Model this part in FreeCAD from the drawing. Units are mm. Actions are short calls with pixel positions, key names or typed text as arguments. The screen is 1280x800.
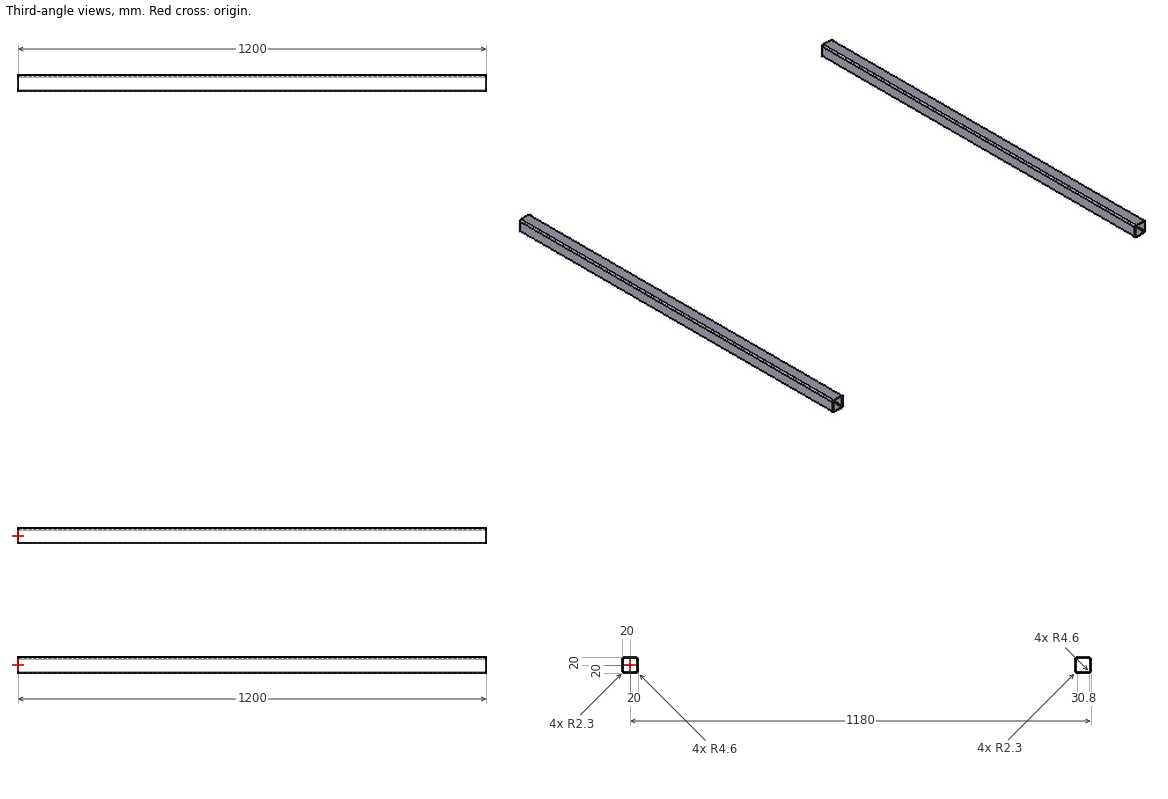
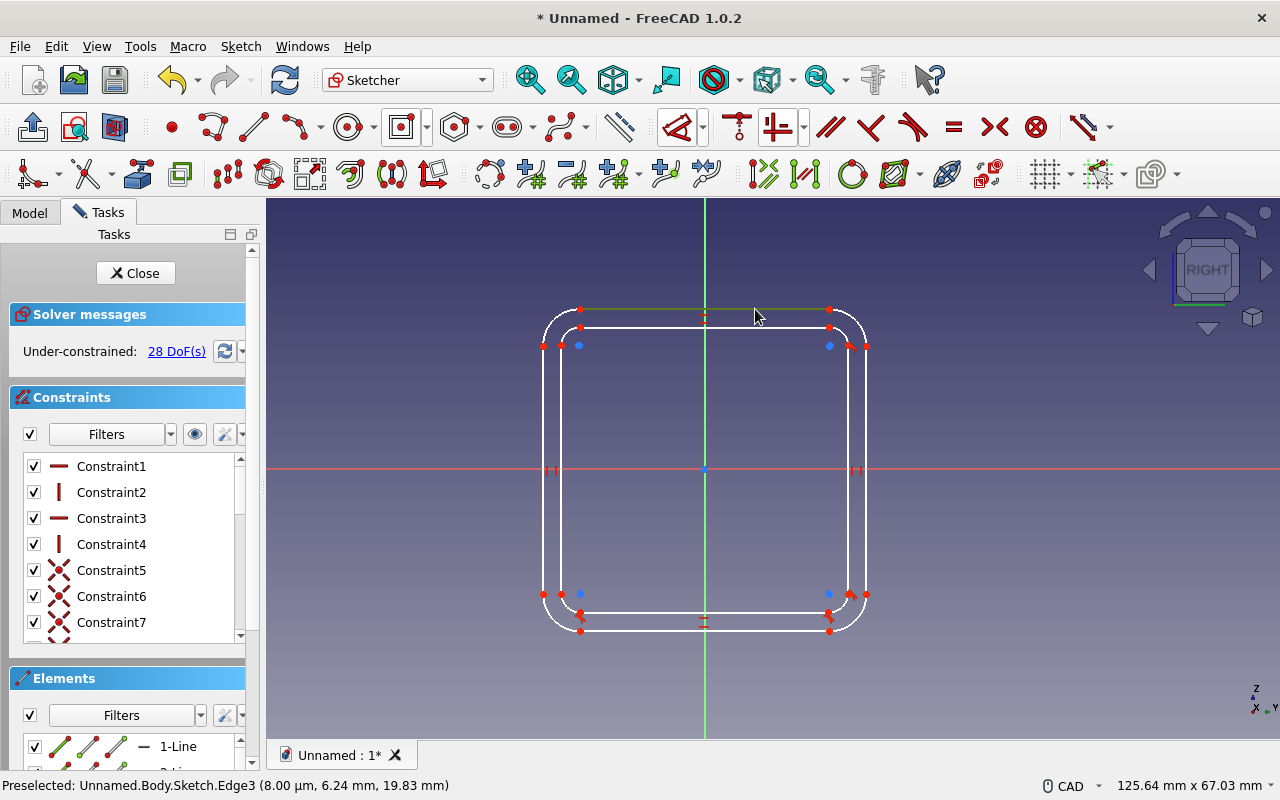
click(862, 330)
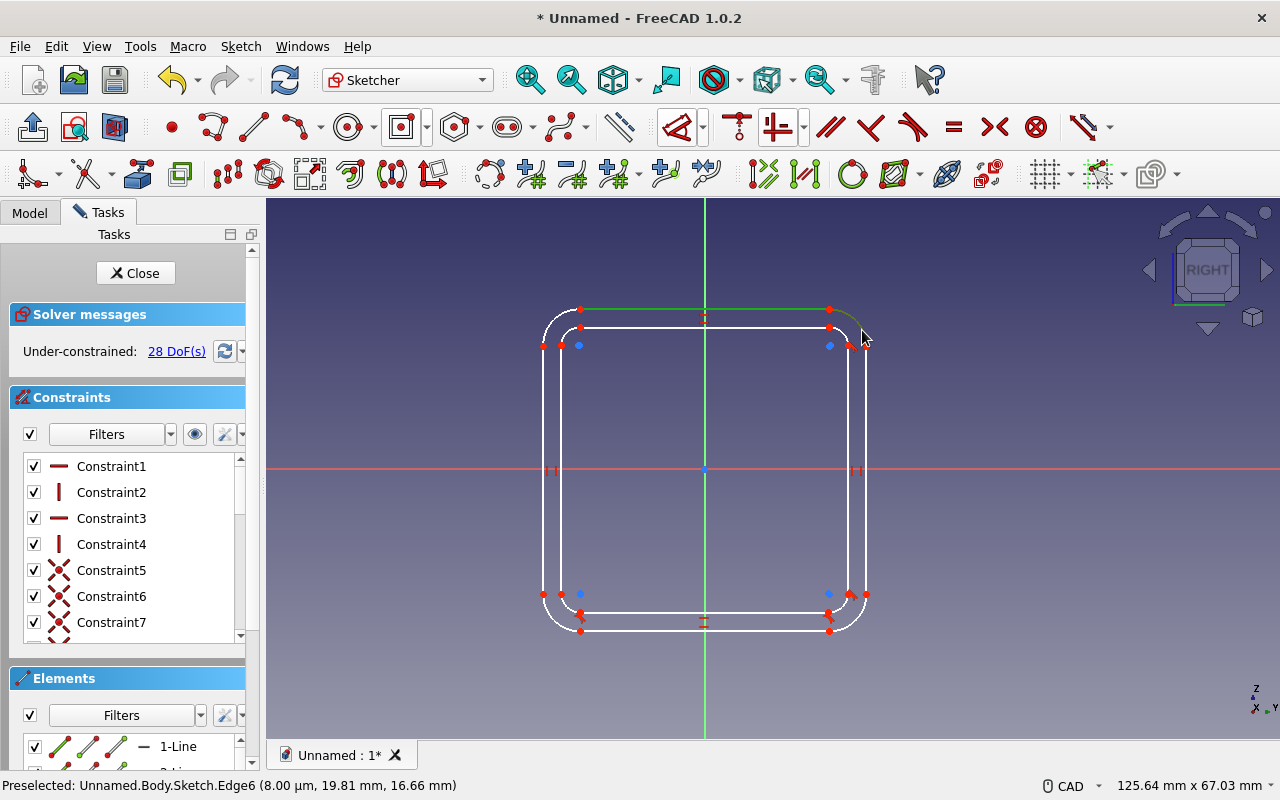
click(913, 128)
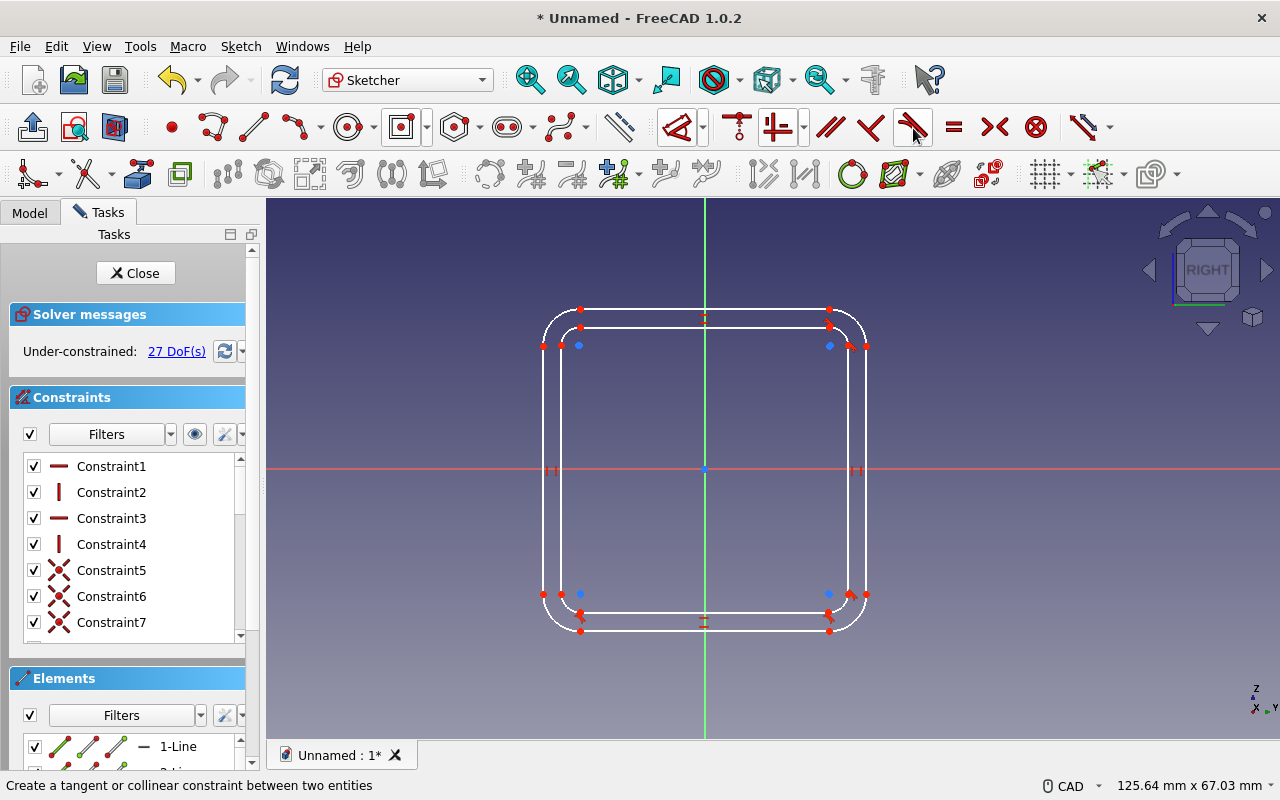
click(755, 309)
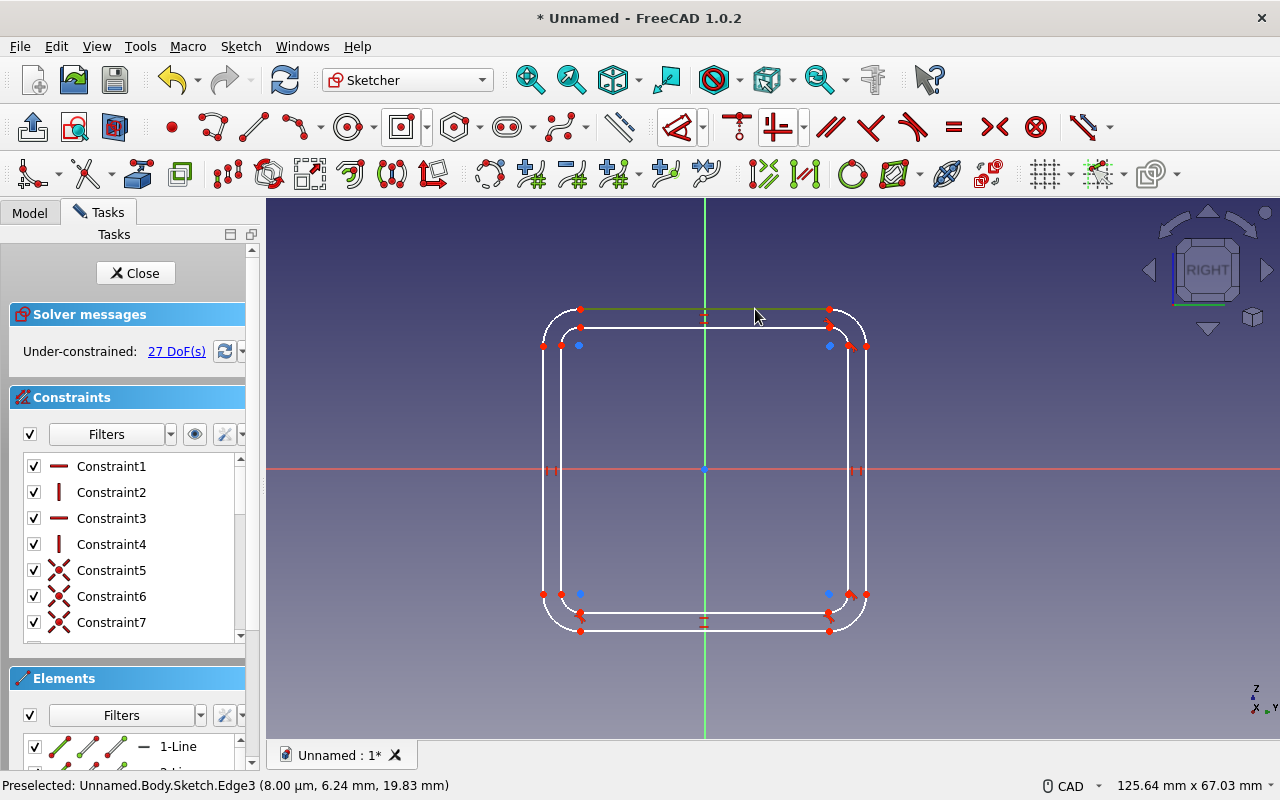
click(563, 313)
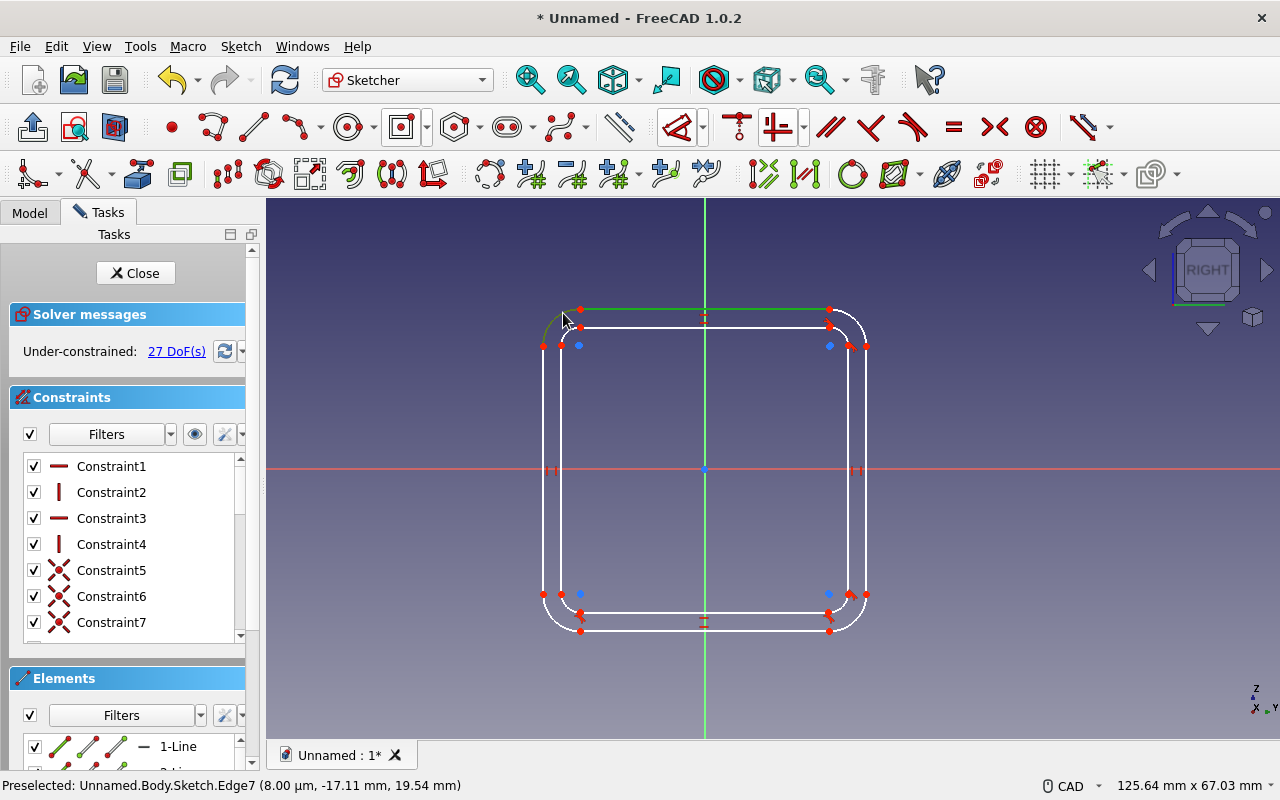
click(913, 128)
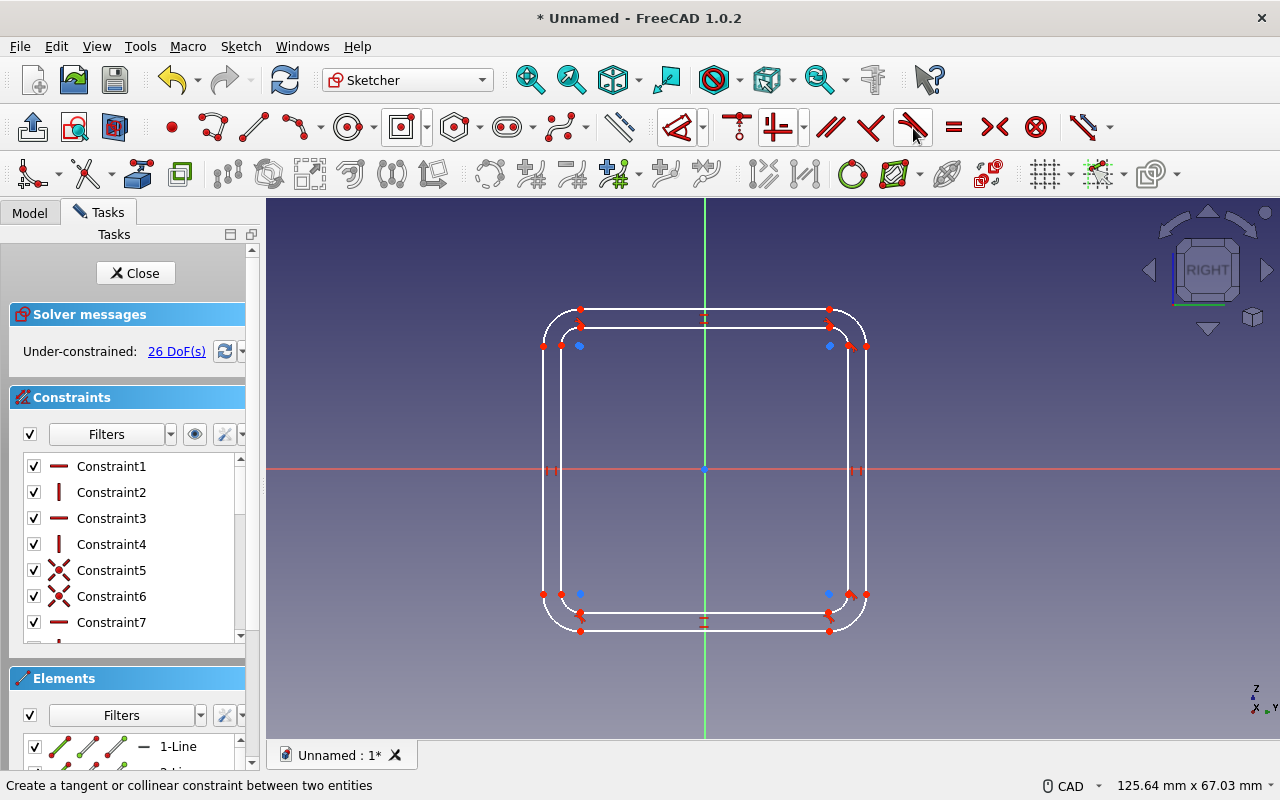
click(543, 421)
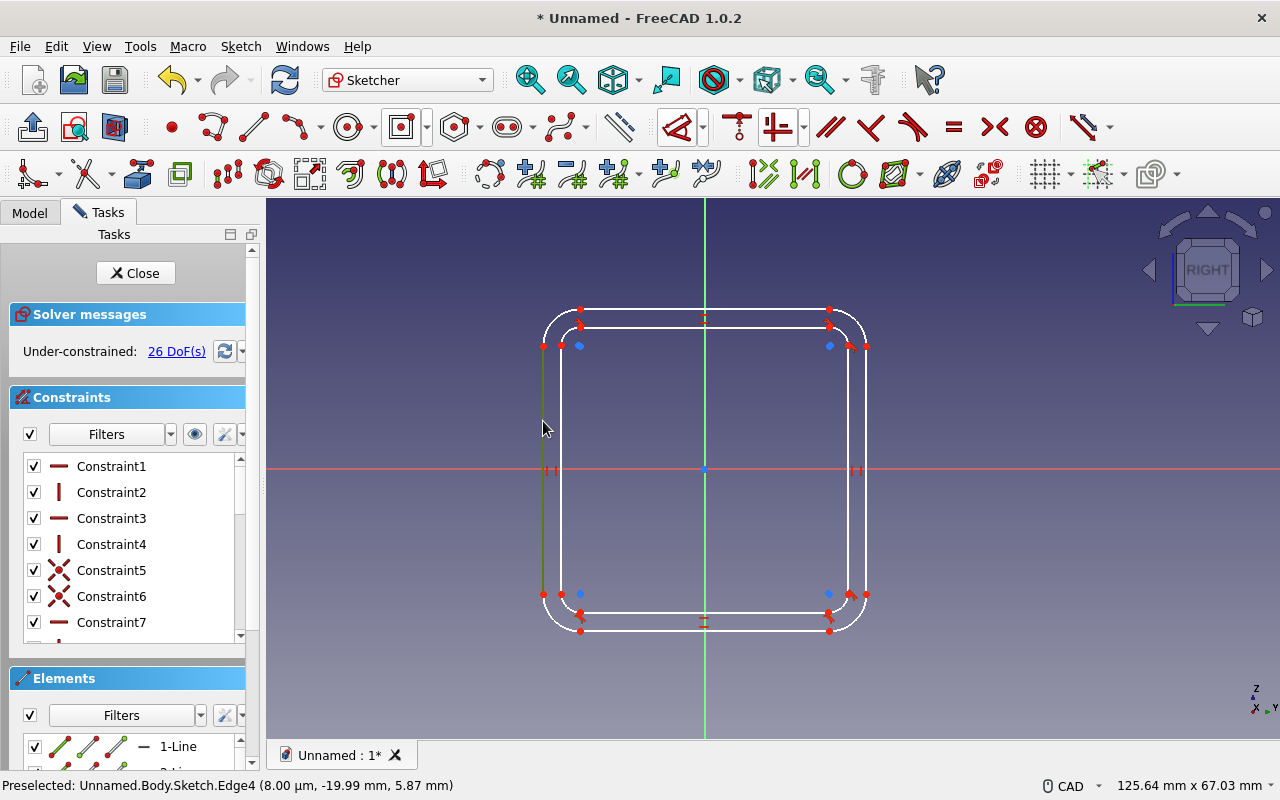
click(564, 313)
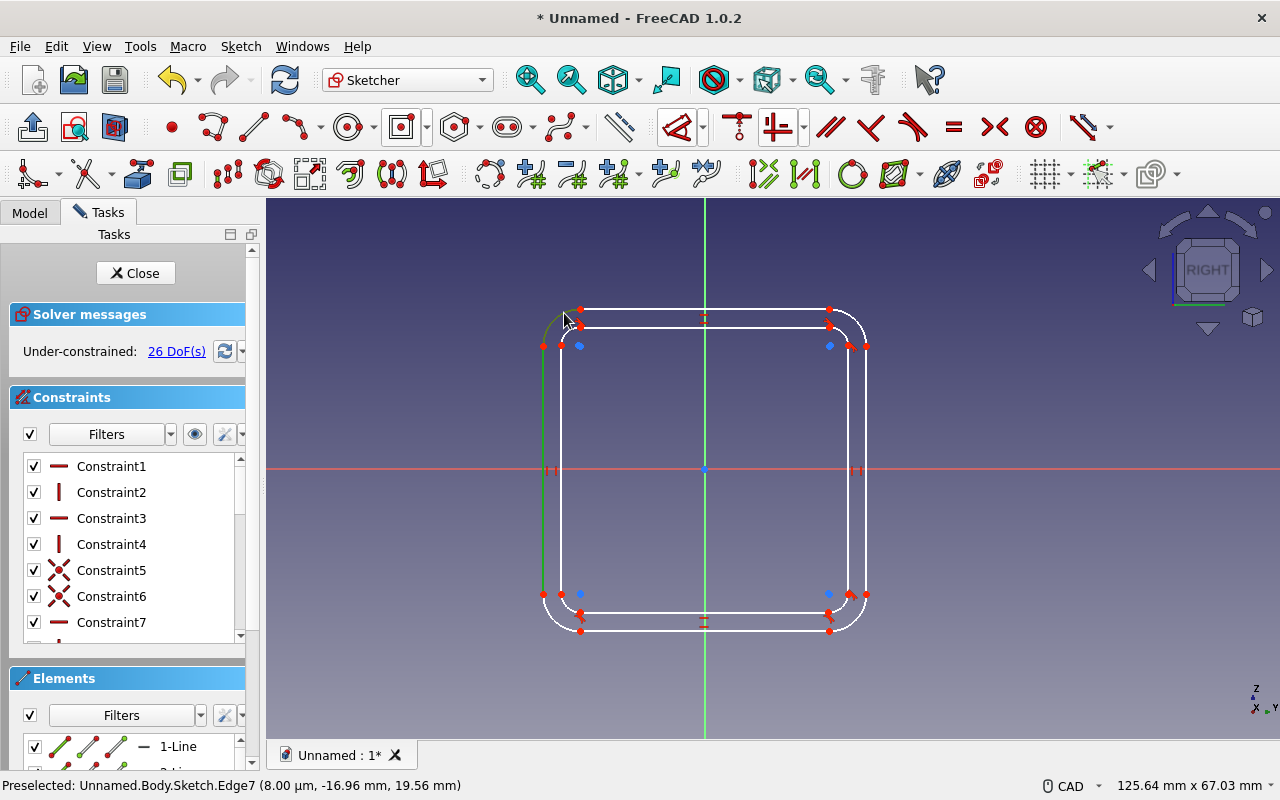
key(t)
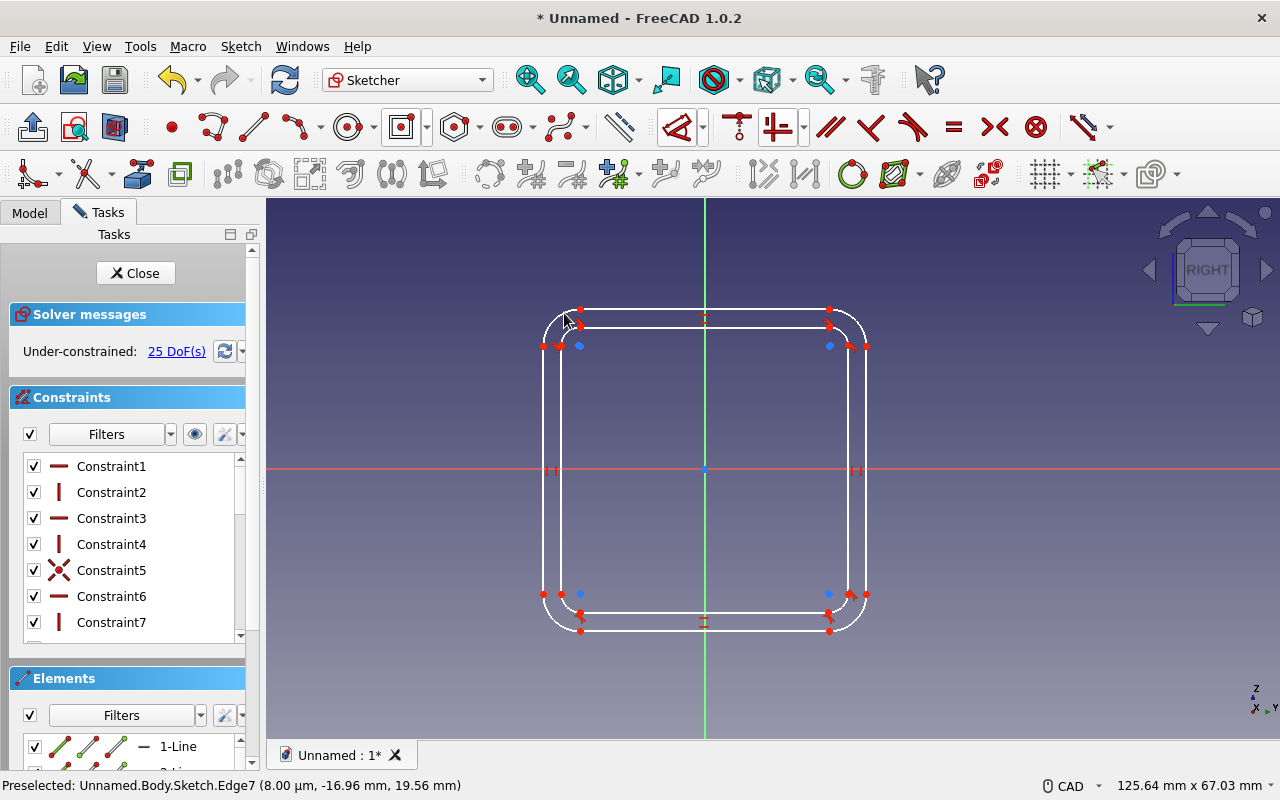
click(543, 421)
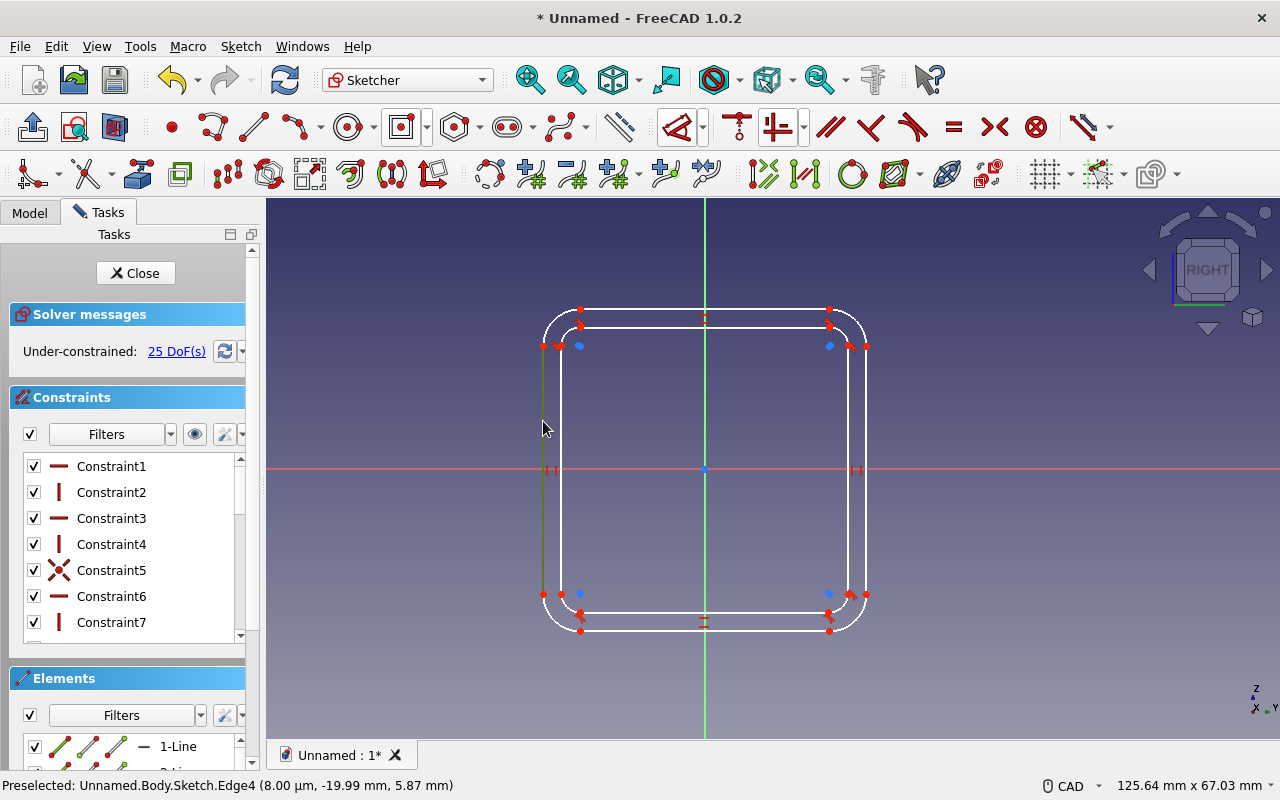
click(547, 611)